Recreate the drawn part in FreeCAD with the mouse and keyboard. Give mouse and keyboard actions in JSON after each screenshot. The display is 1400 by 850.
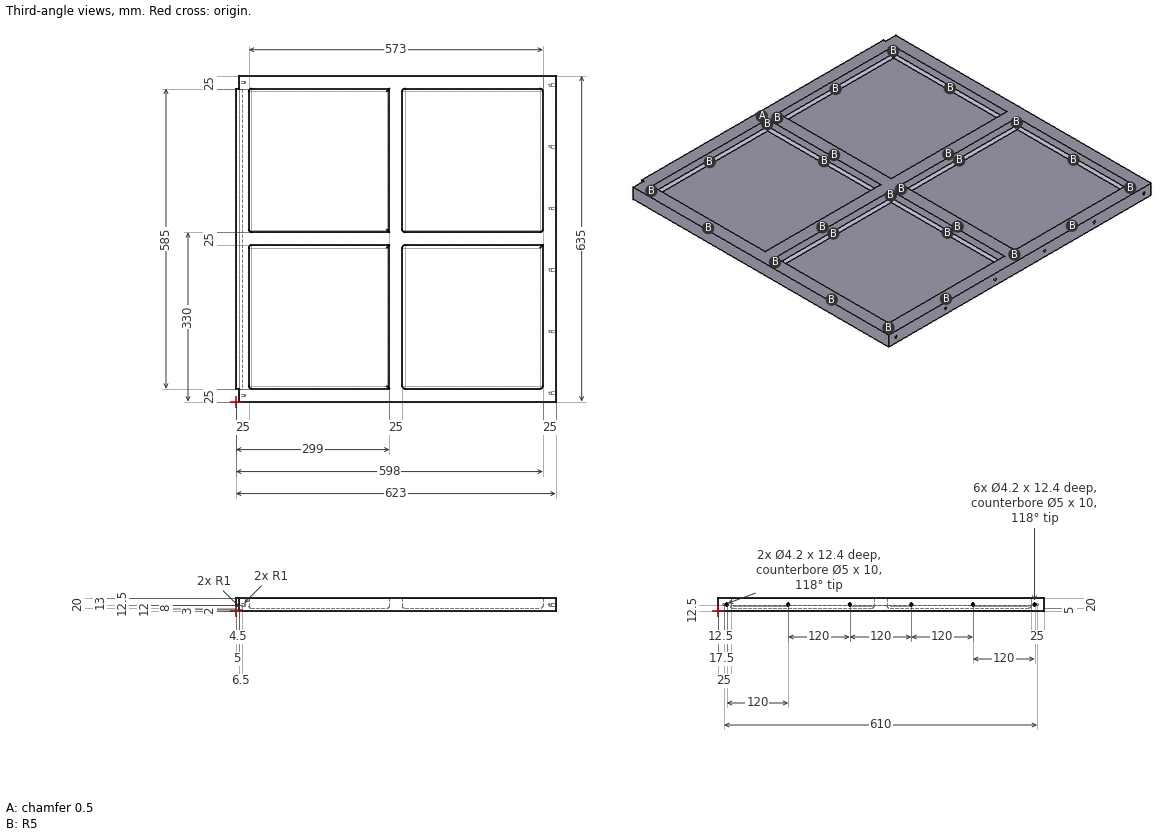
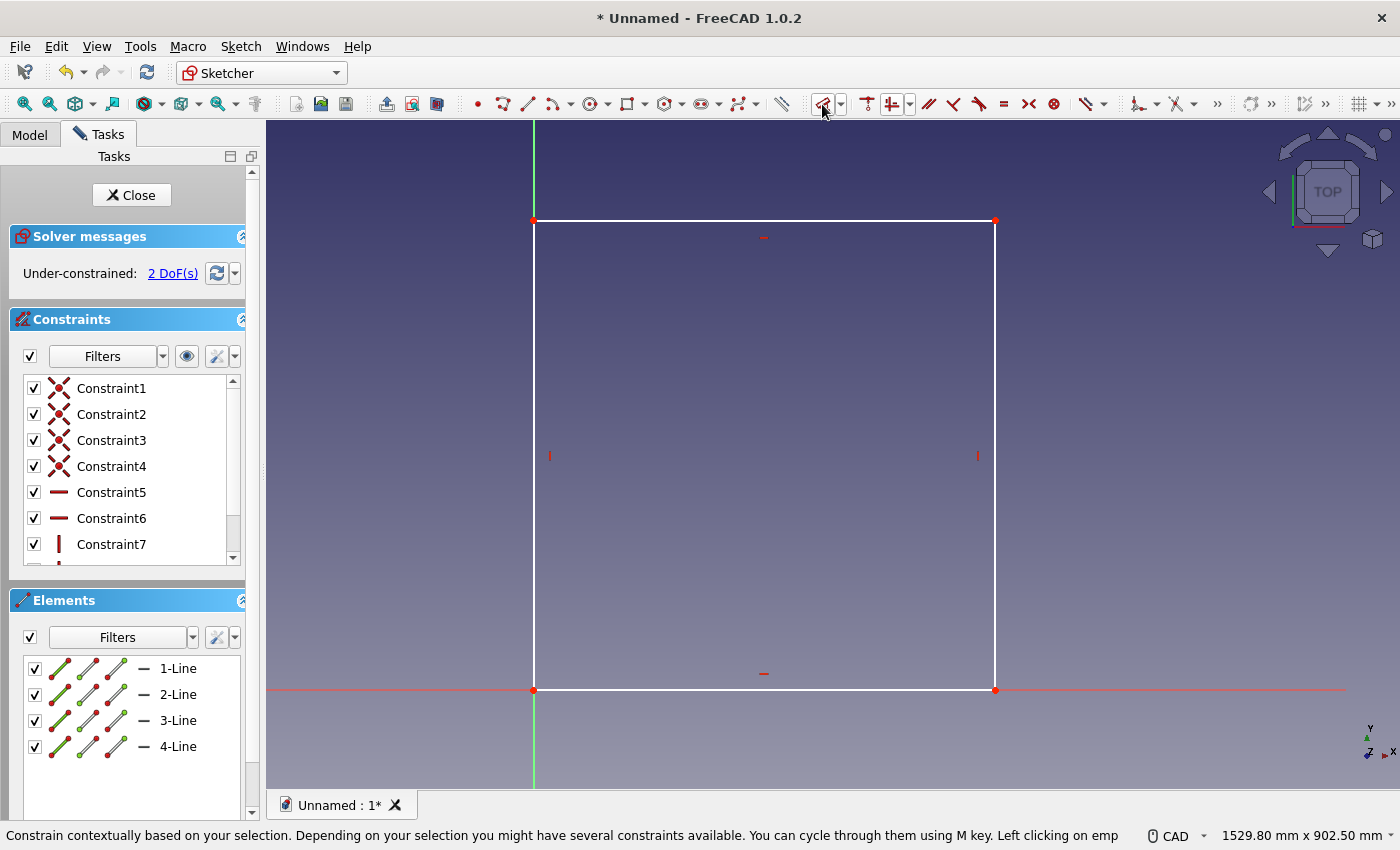
{"action": "left_click", "coordinate": [672, 690]}
{"action": "left_click", "coordinate": [764, 724]}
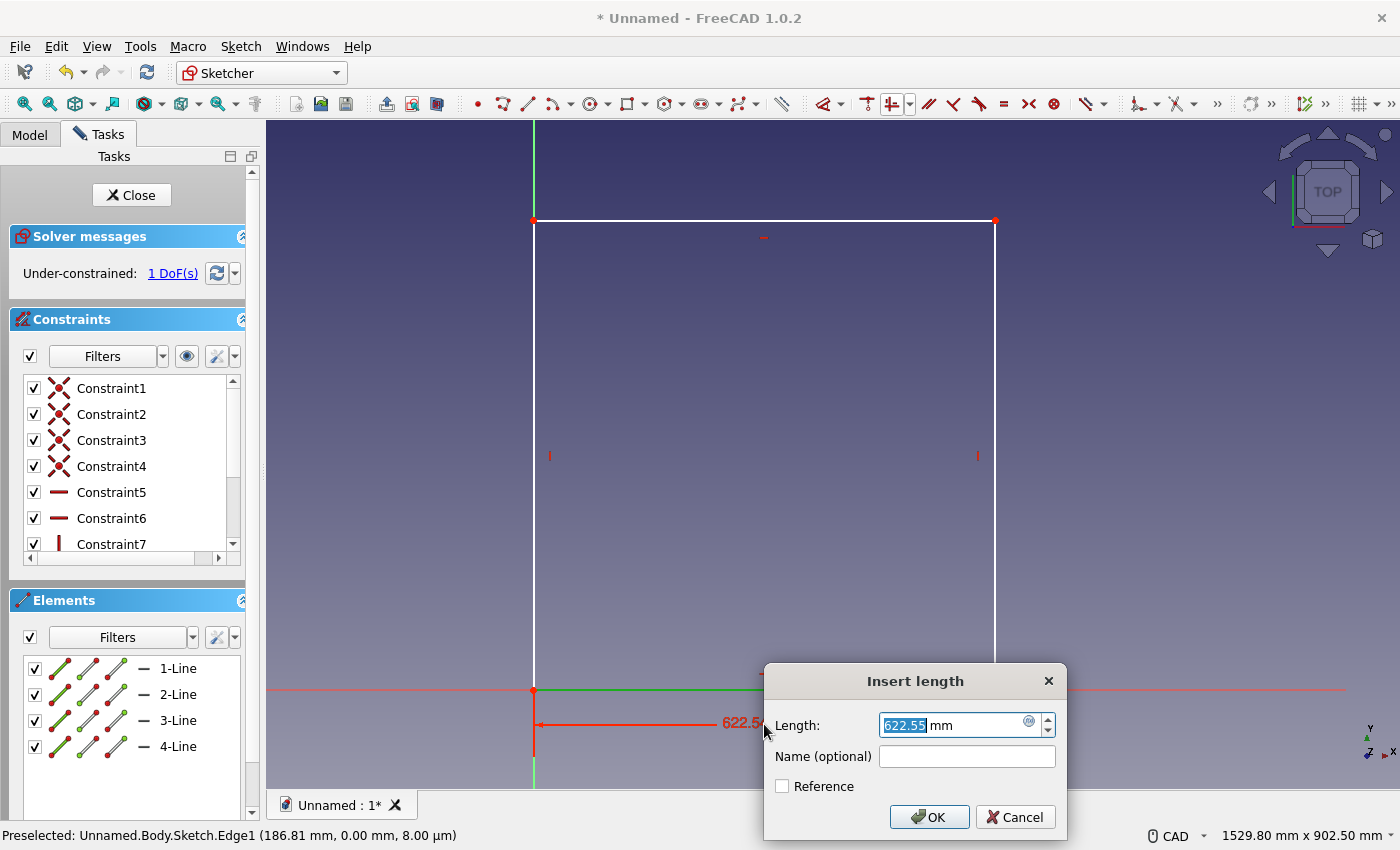
{"action": "type", "text": "623"}
{"action": "key", "text": "Return"}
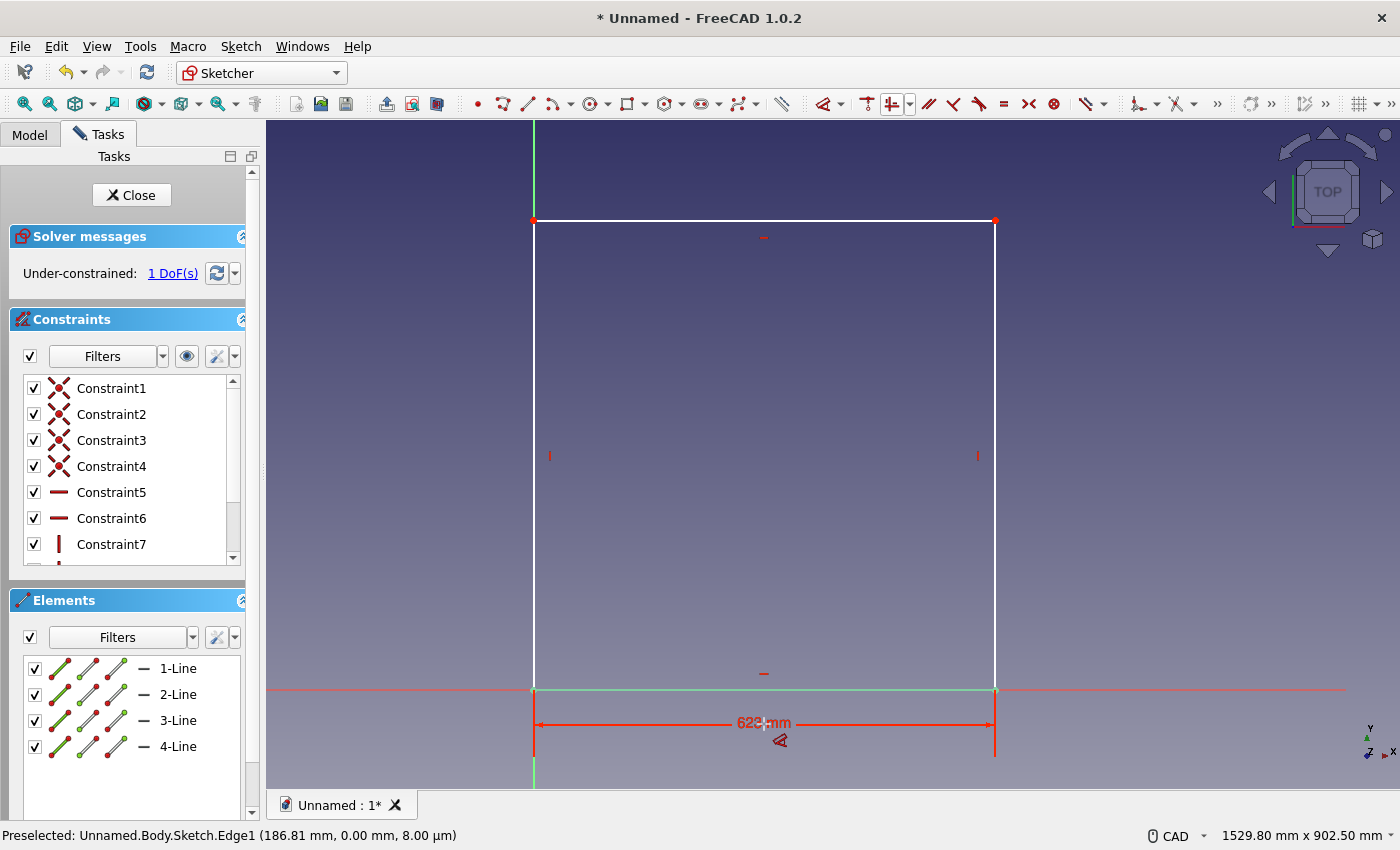
{"action": "left_click", "coordinate": [995, 550]}
{"action": "left_click", "coordinate": [1029, 456]}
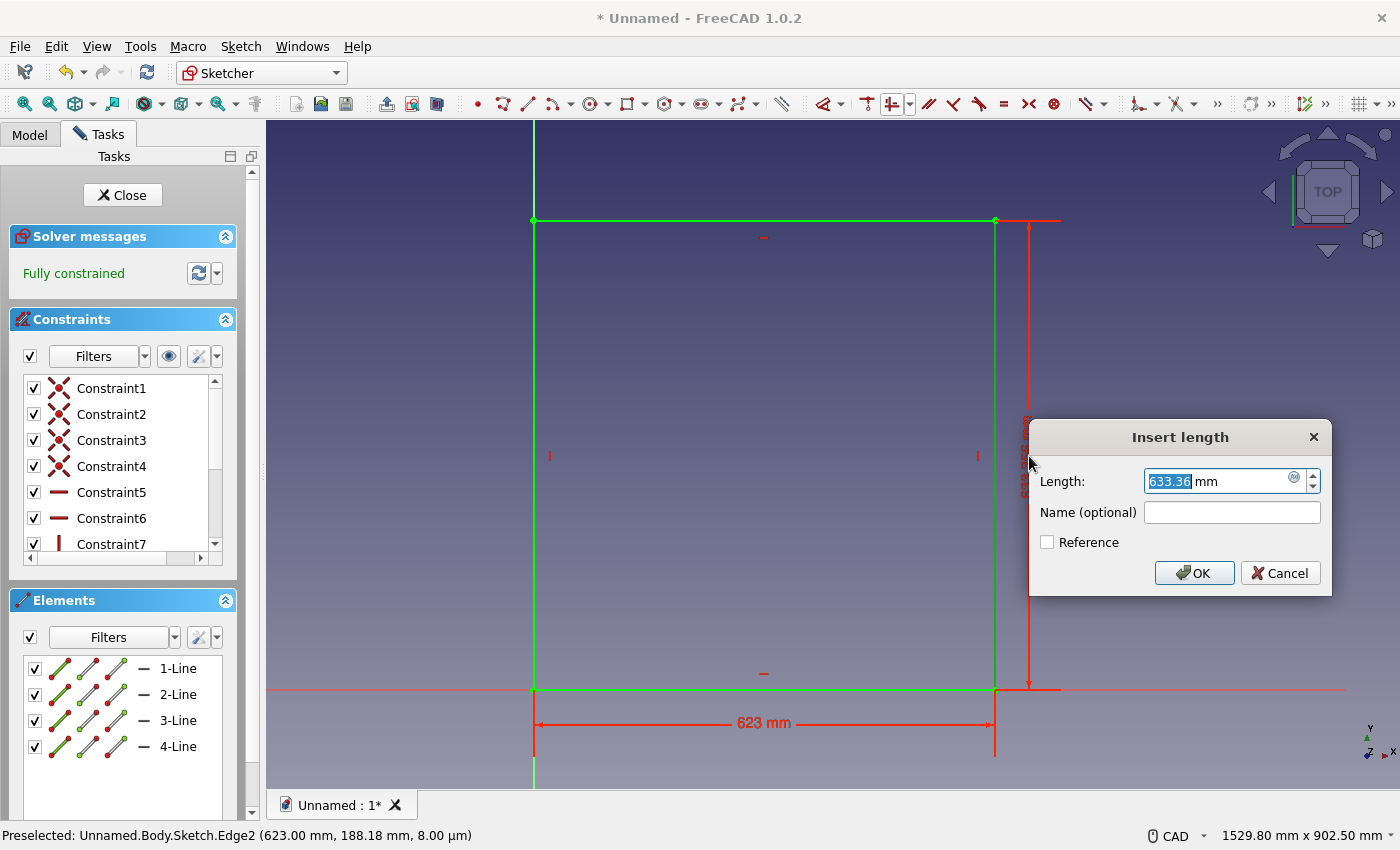
{"action": "type", "text": "635"}
{"action": "key", "text": "Return"}
{"action": "key", "text": "Escape"}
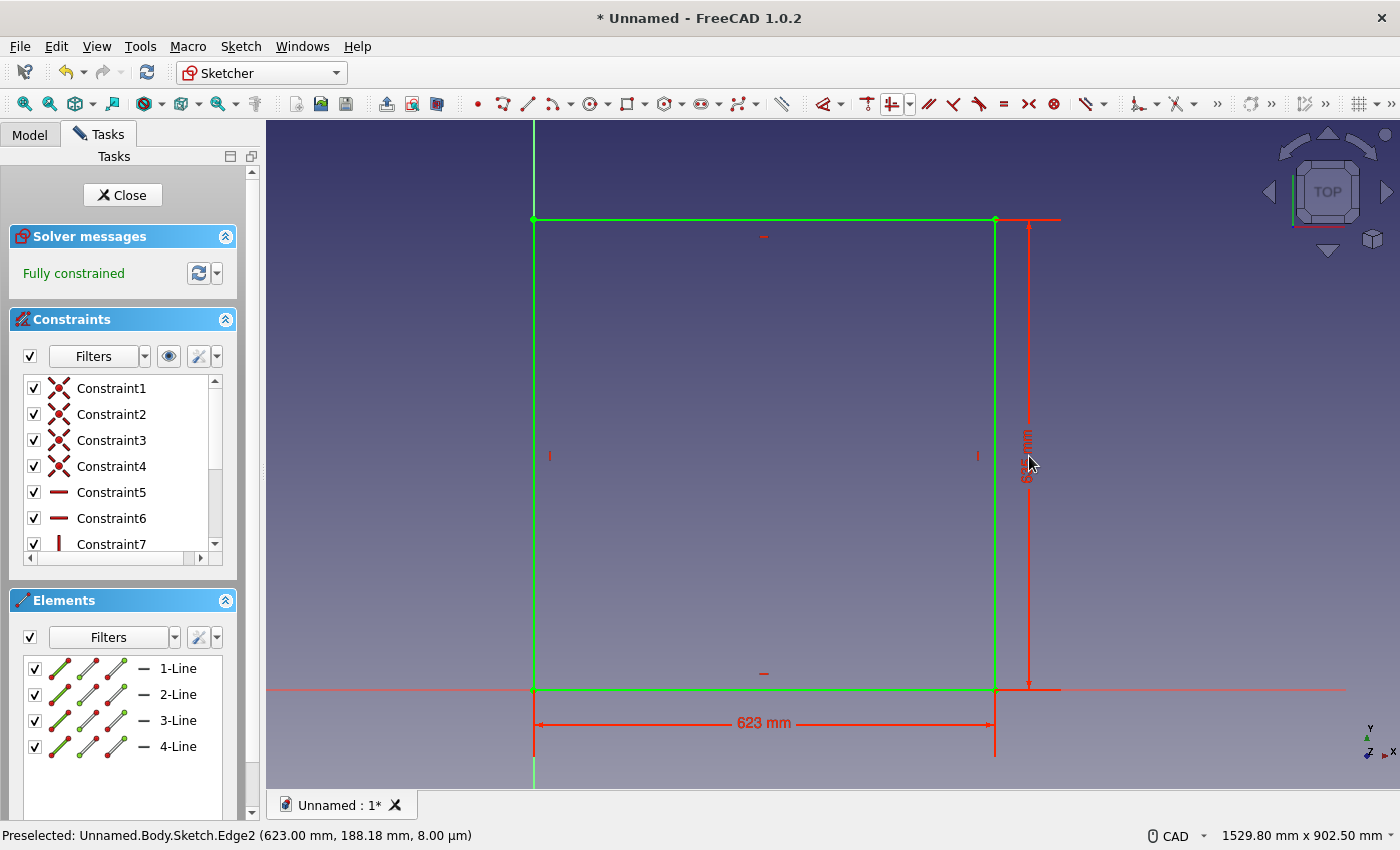
{"action": "left_click", "coordinate": [123, 195]}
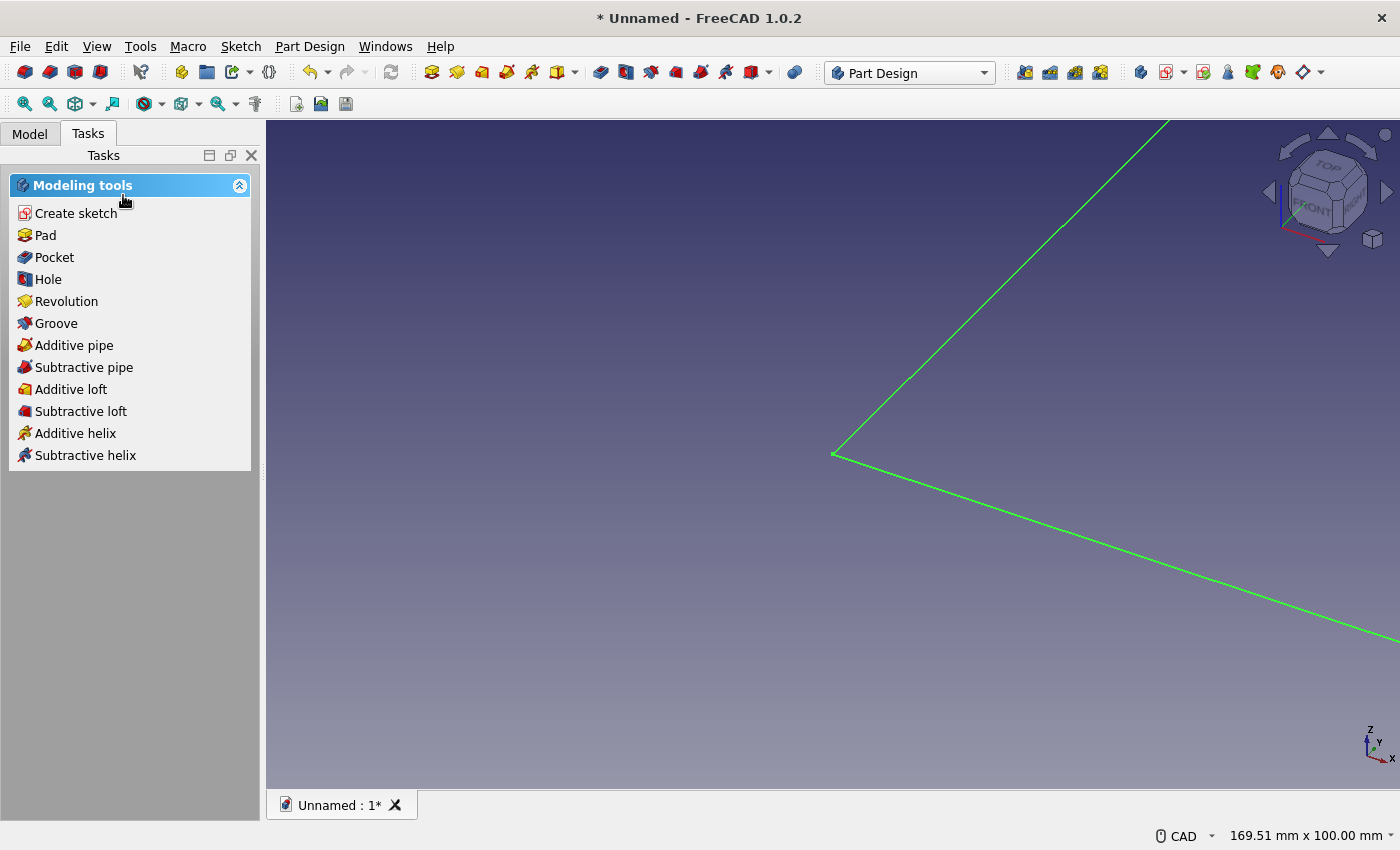
{"action": "left_click", "coordinate": [432, 72]}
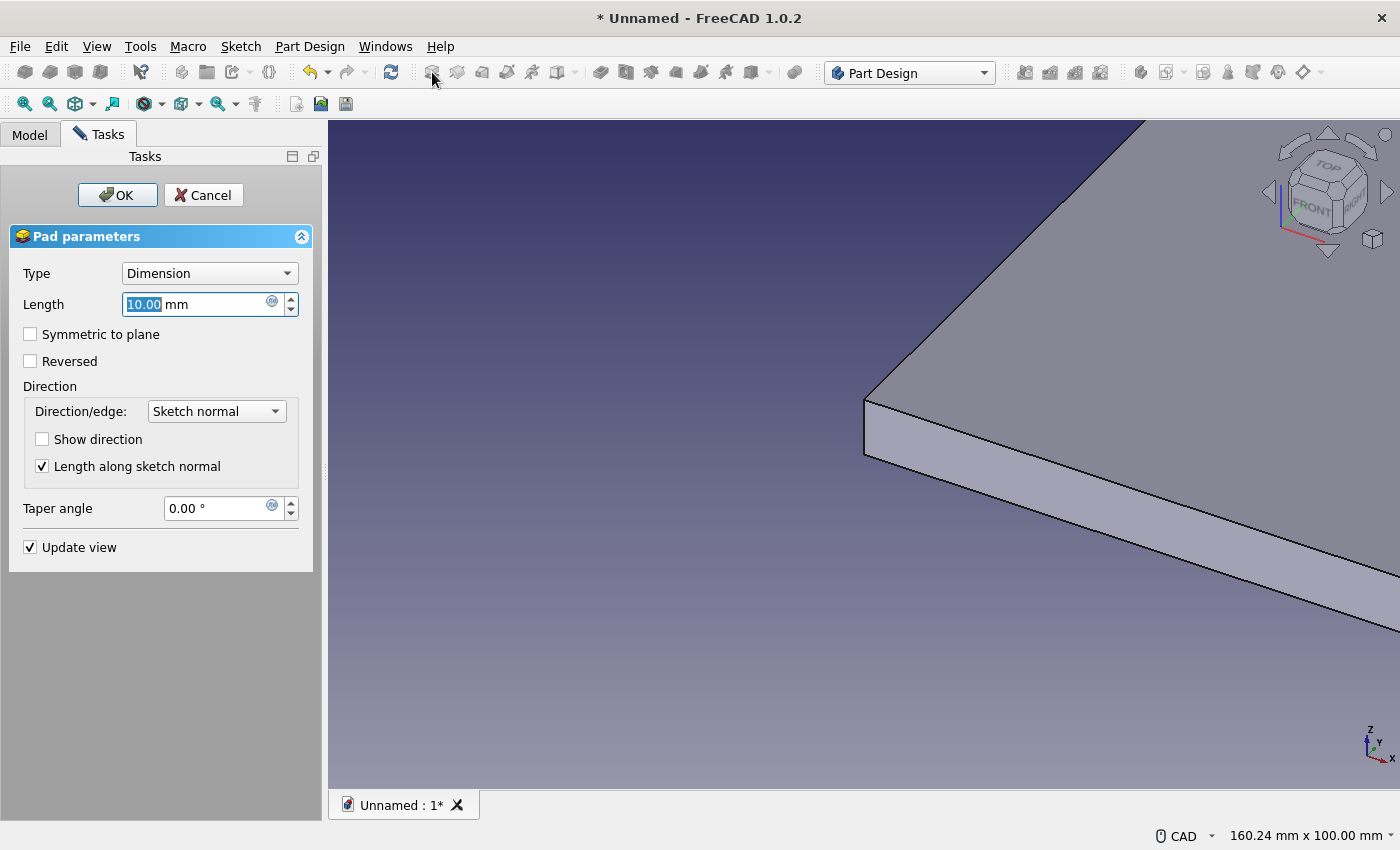
{"action": "type", "text": "5"}
{"action": "key", "text": "Tab"}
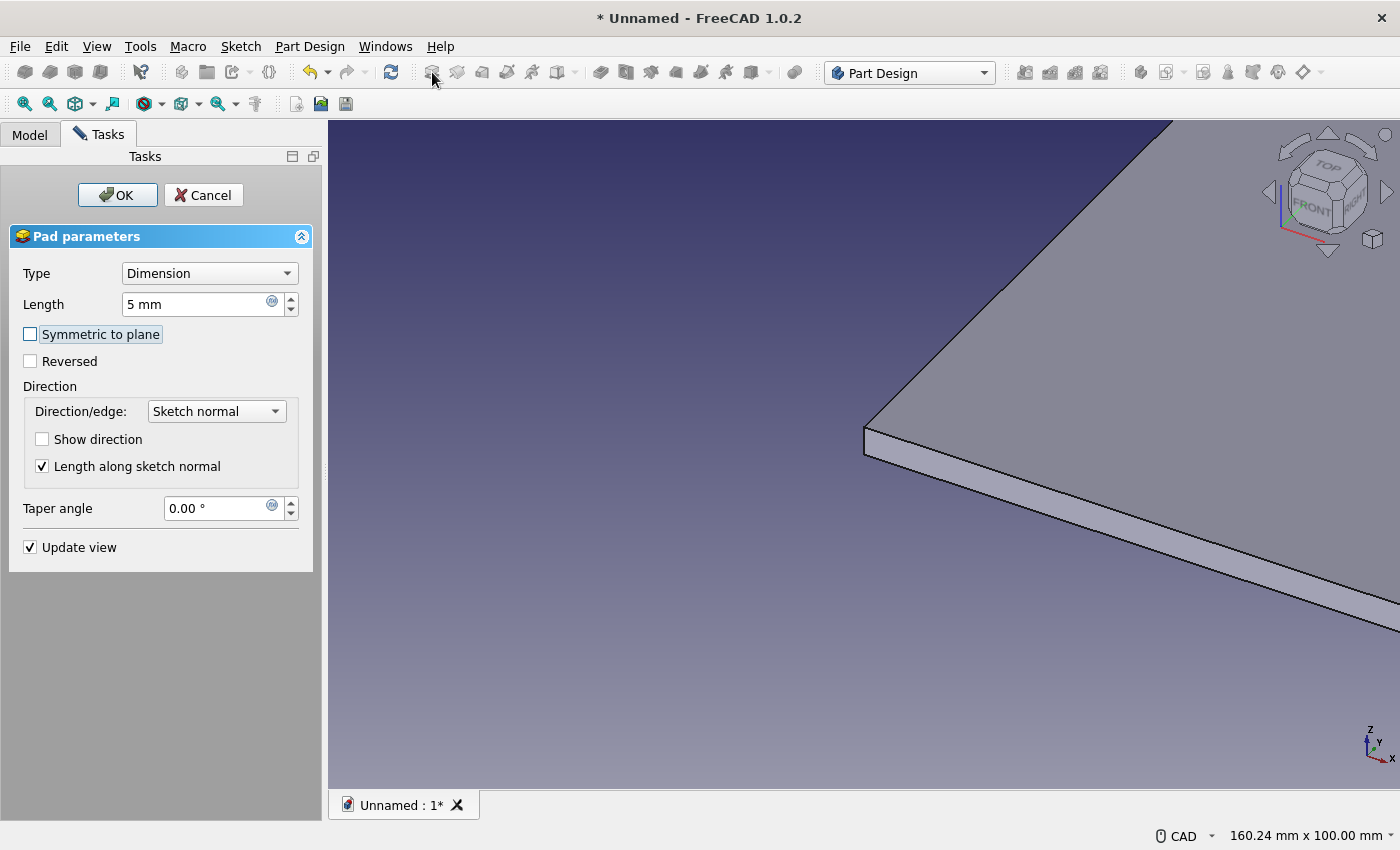
{"action": "left_click", "coordinate": [118, 195]}